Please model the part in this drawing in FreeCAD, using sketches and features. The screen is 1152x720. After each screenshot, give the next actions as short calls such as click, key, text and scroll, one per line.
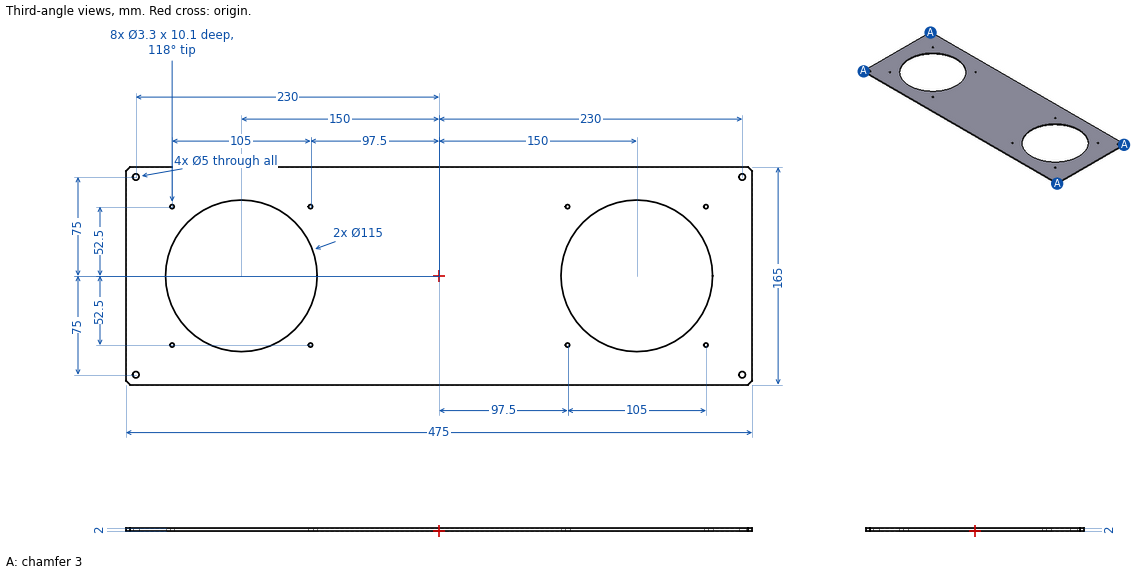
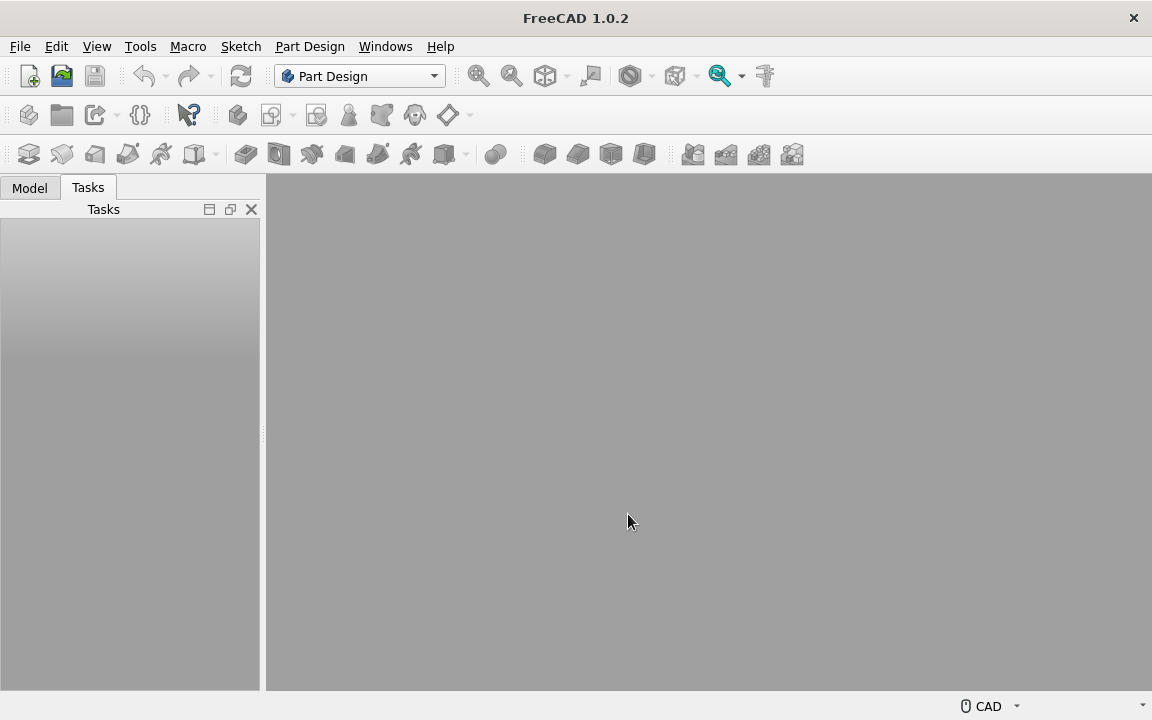
key(ctrl+n)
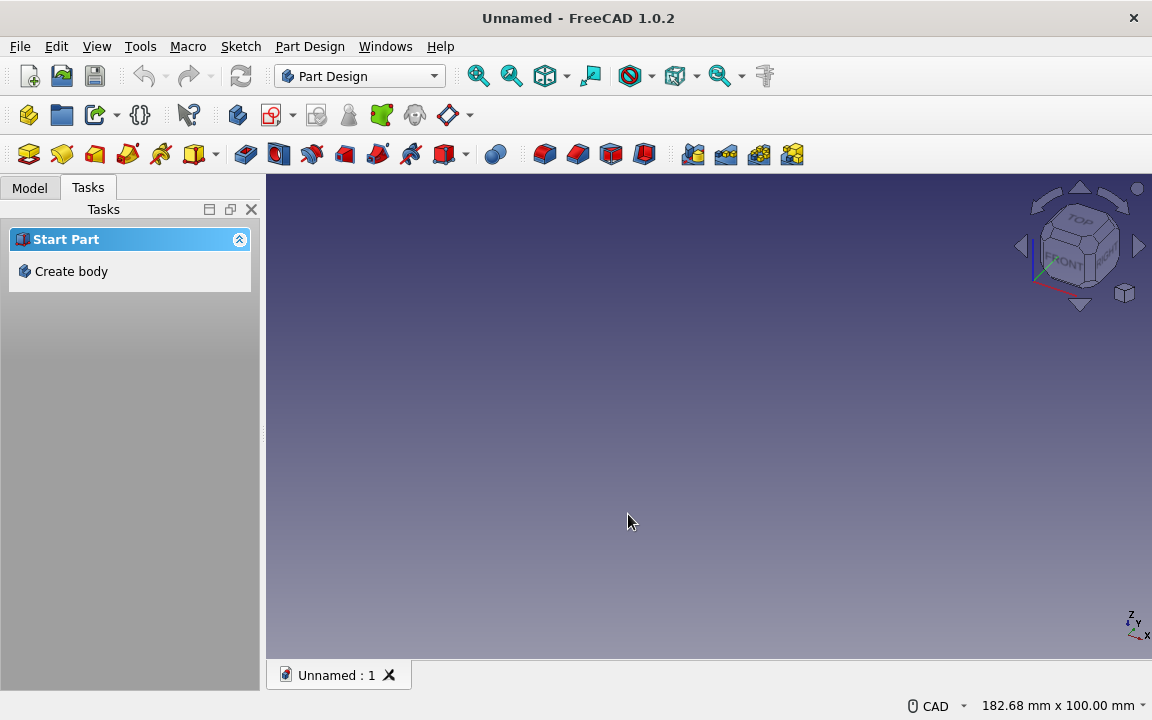
click(270, 116)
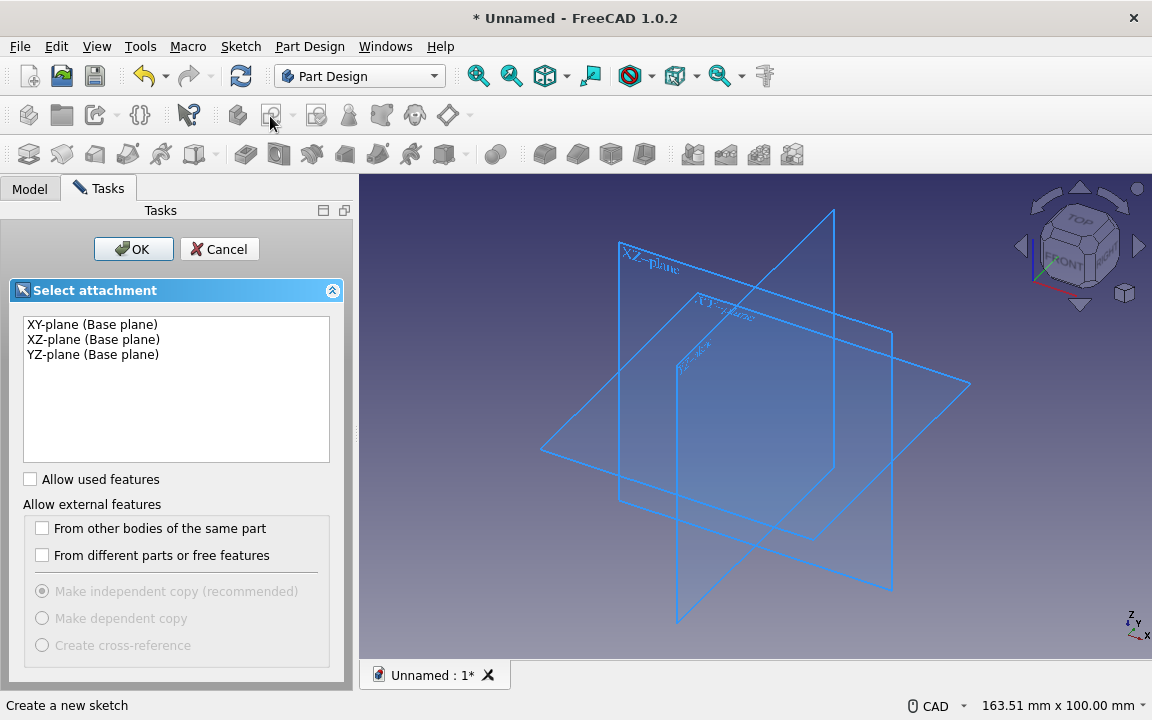
click(84, 324)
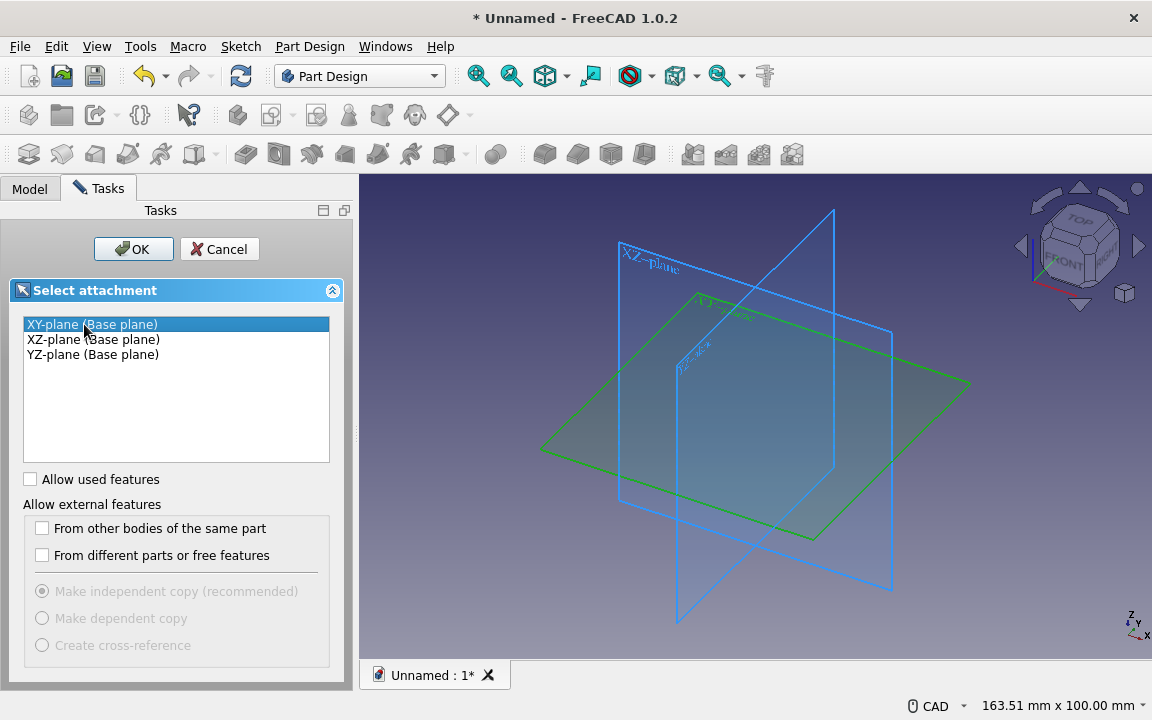
click(134, 249)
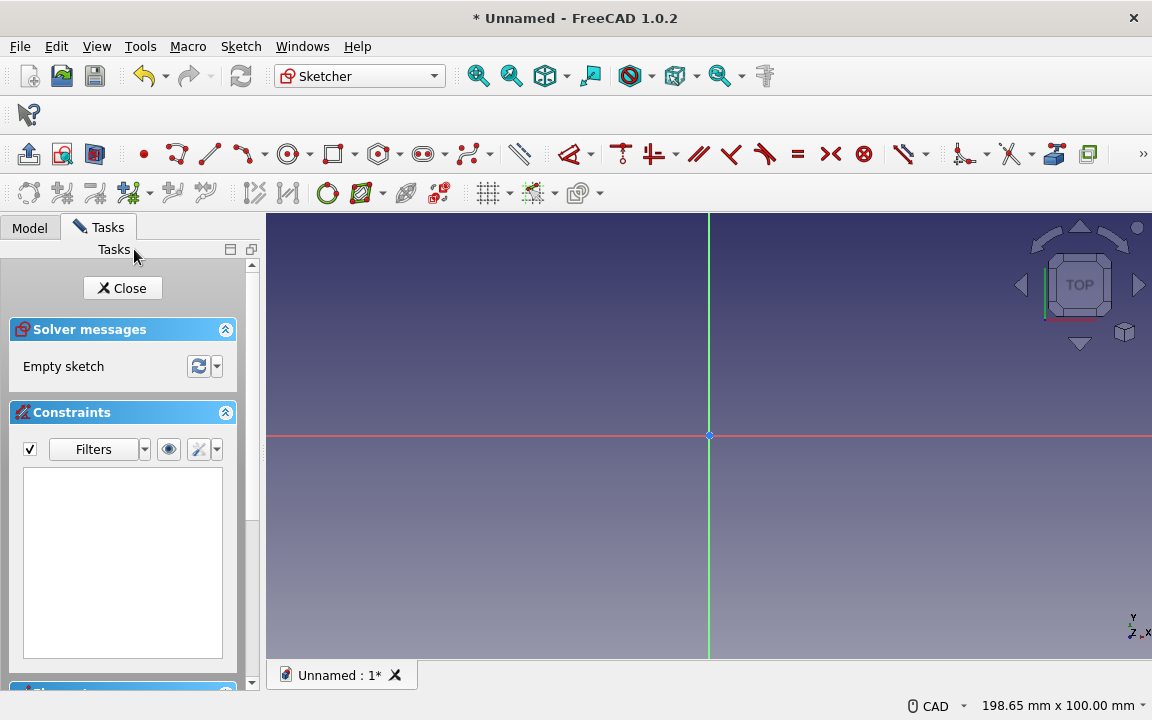
scroll(618, 436, down, 7)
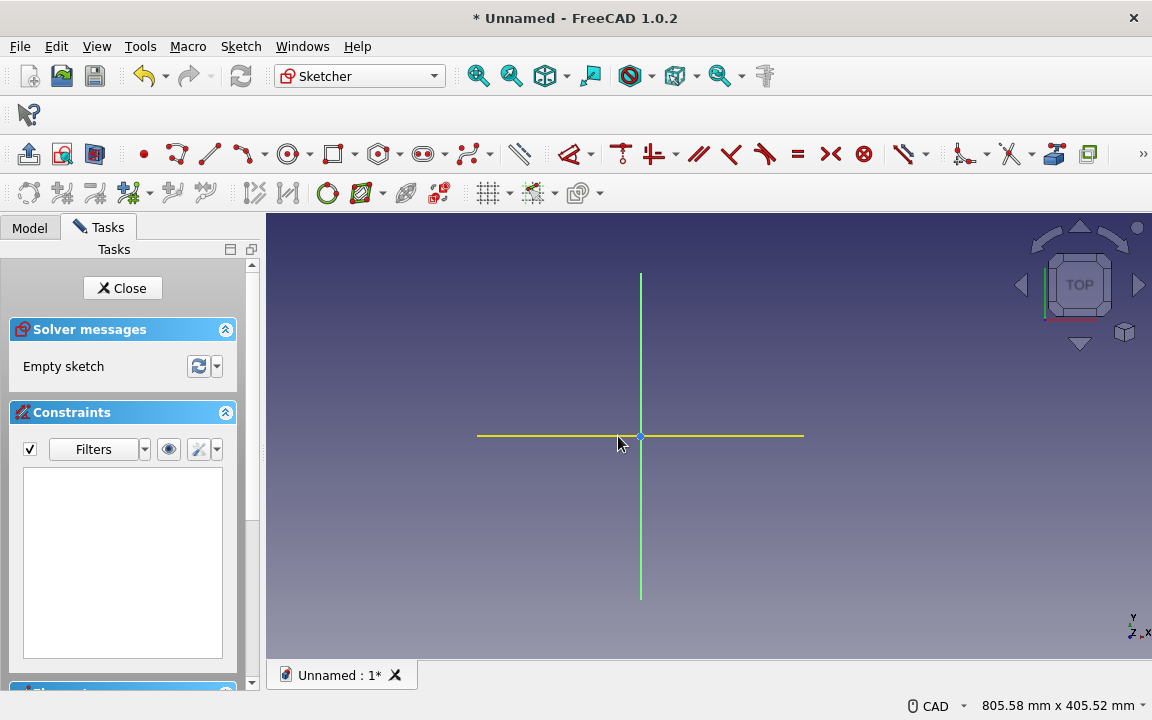
key(g)
key(v)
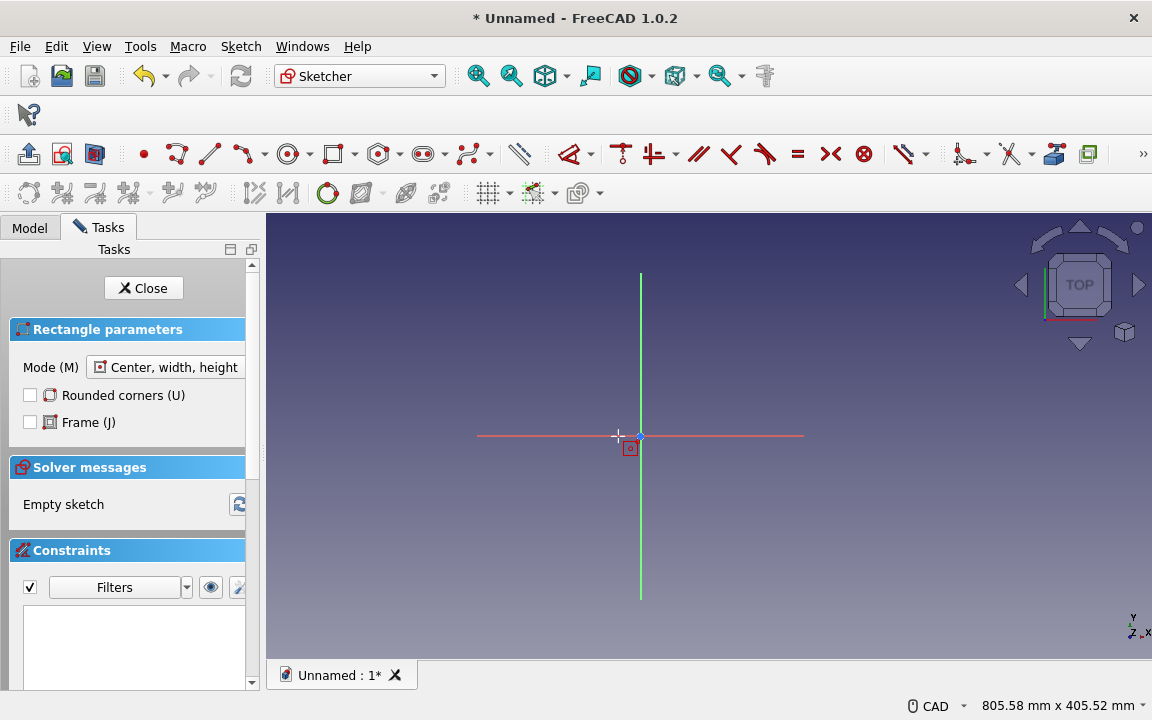
click(641, 436)
move(902, 346)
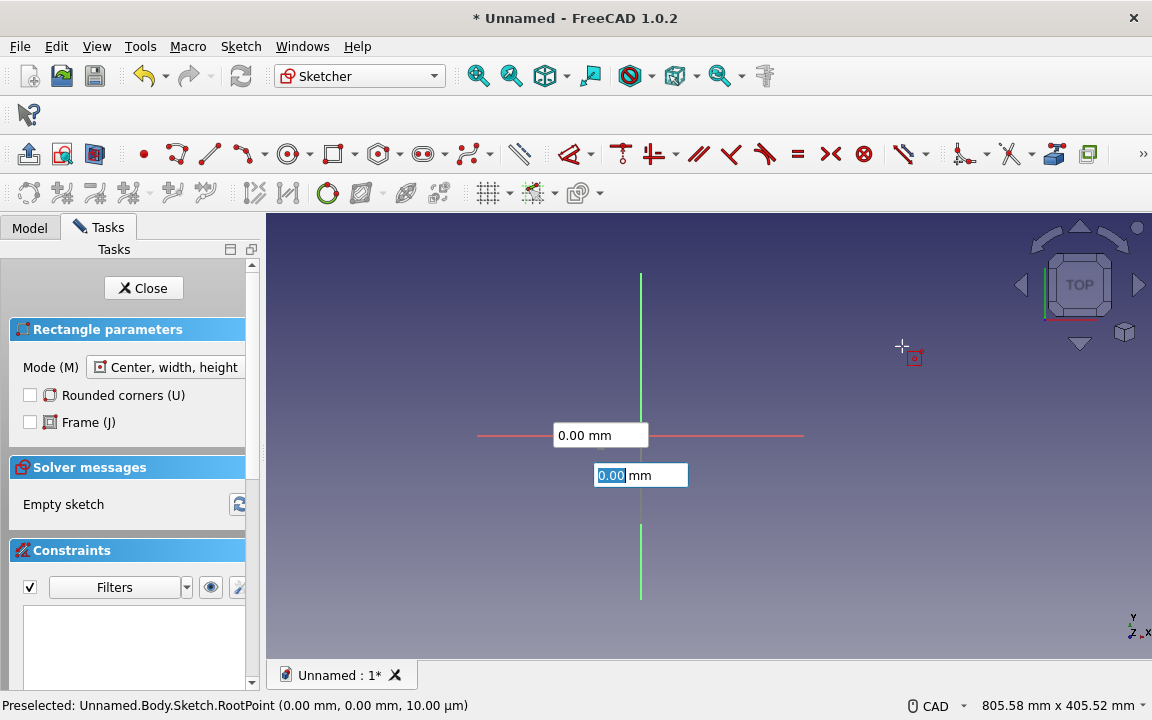
text(475)
key(Tab)
text(165)
key(Return)
key(Escape)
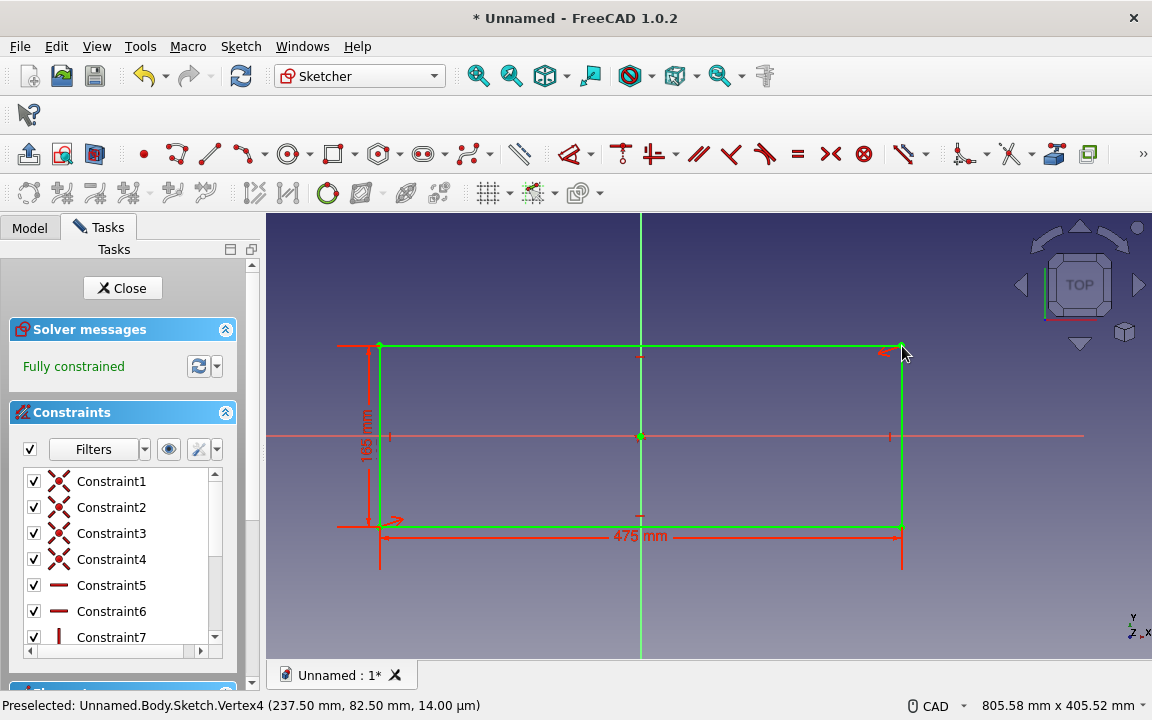
click(123, 288)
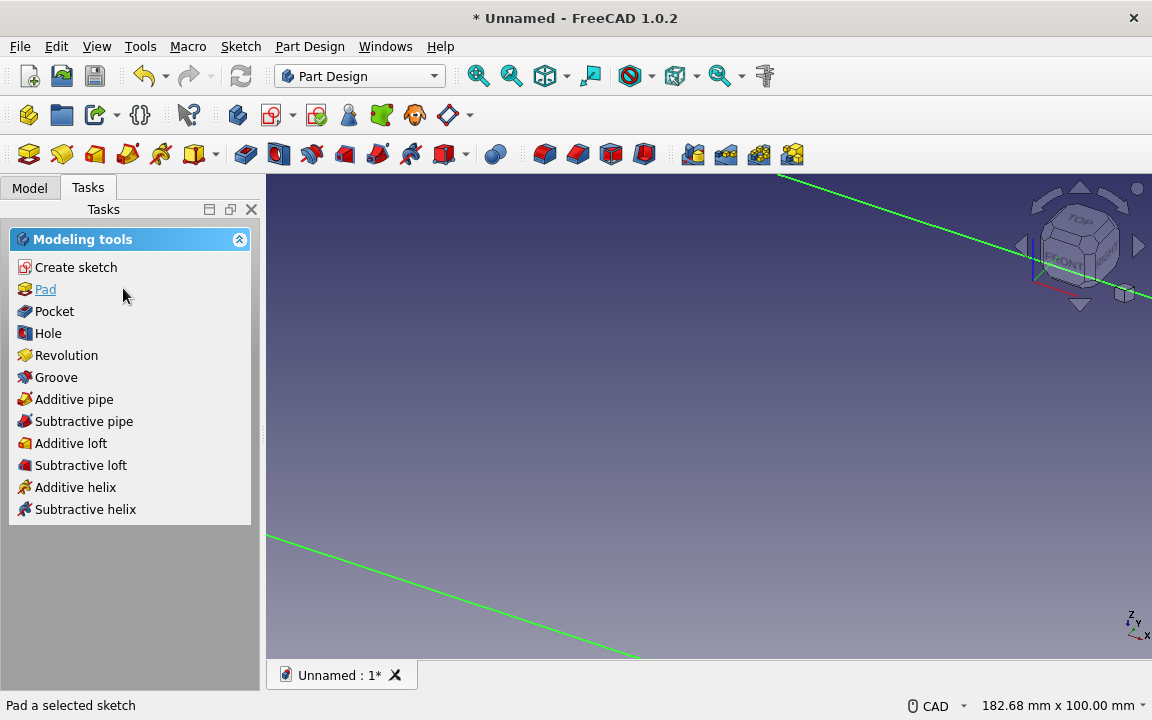
click(29, 154)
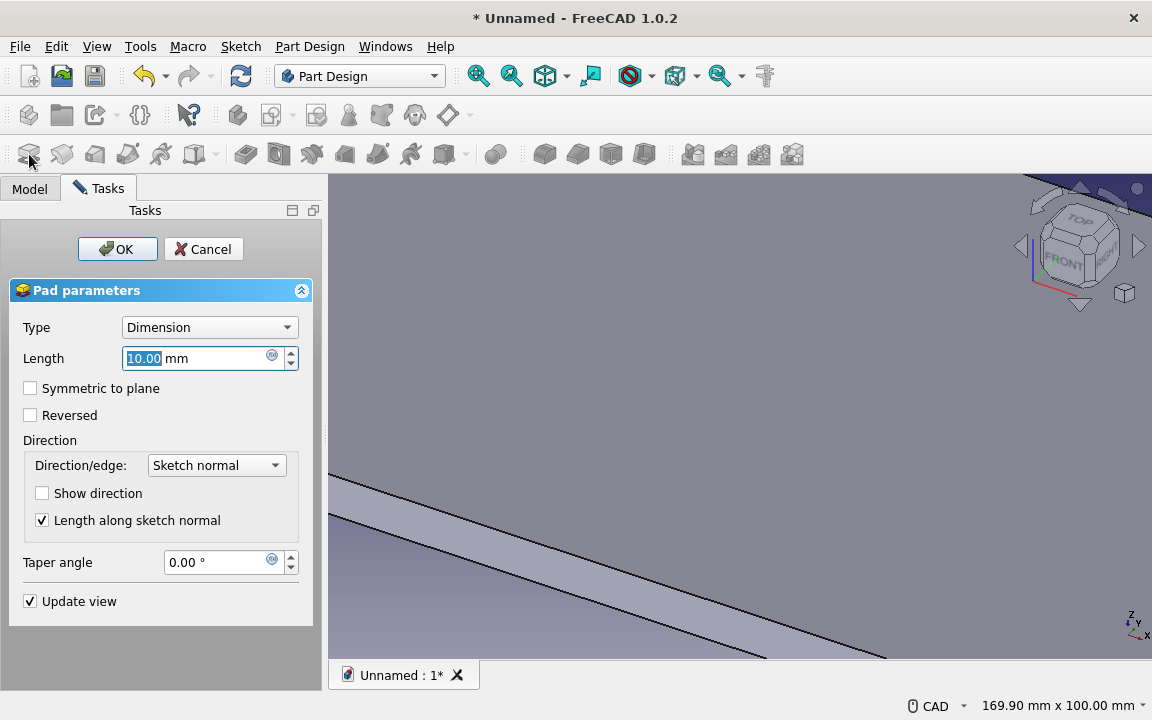
text(2)
key(Tab)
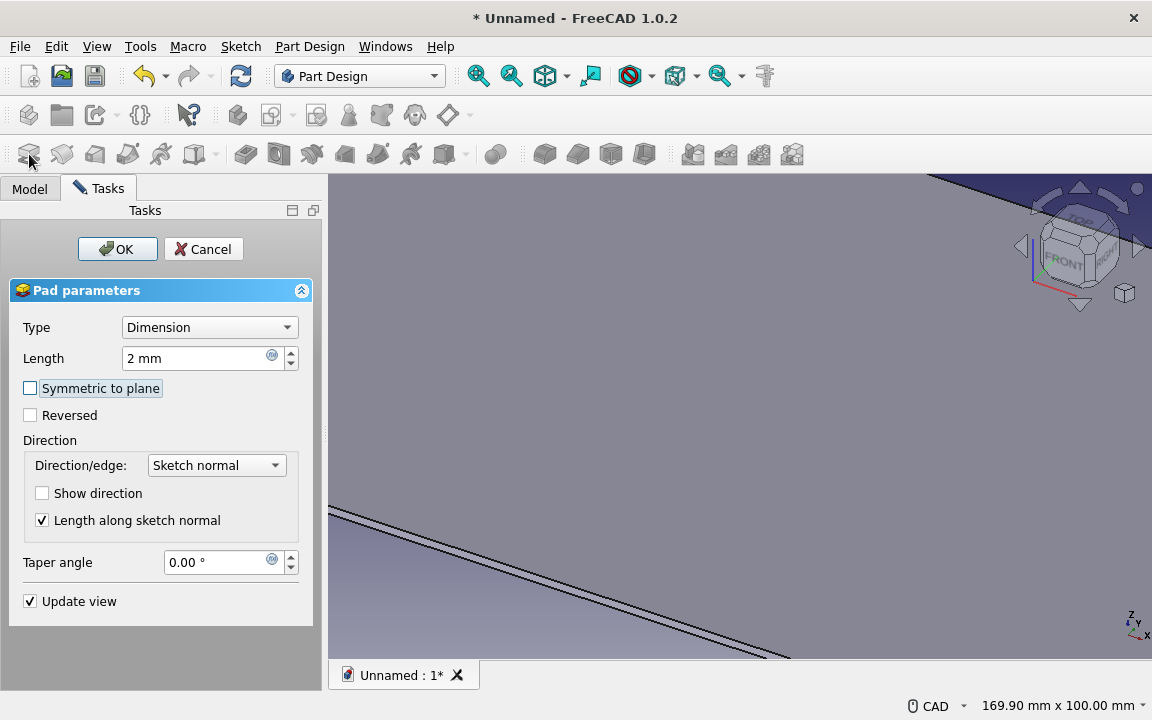
click(118, 249)